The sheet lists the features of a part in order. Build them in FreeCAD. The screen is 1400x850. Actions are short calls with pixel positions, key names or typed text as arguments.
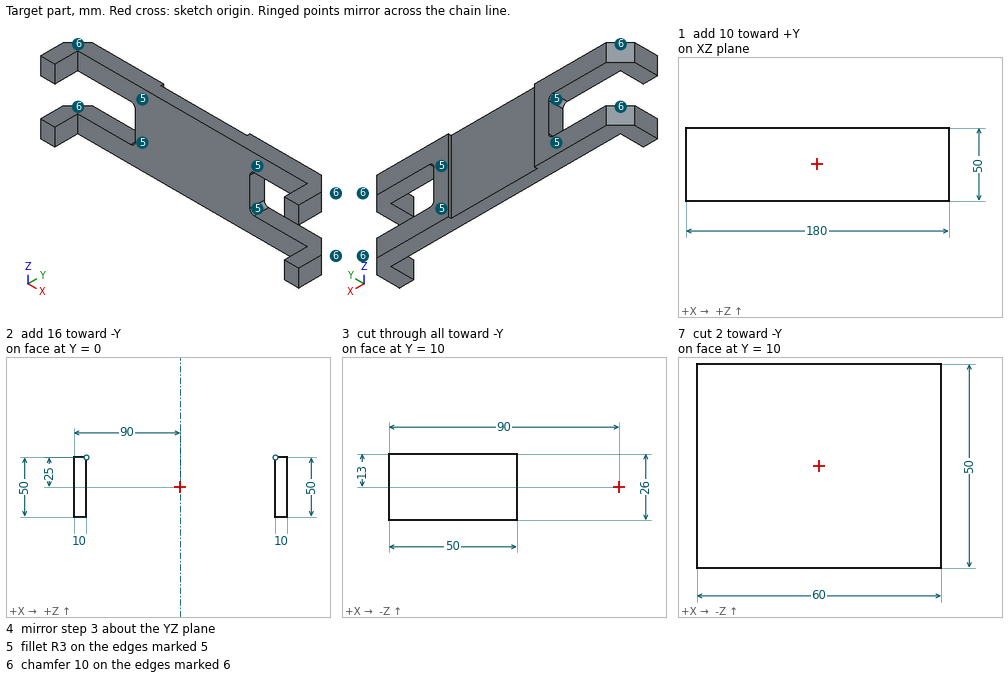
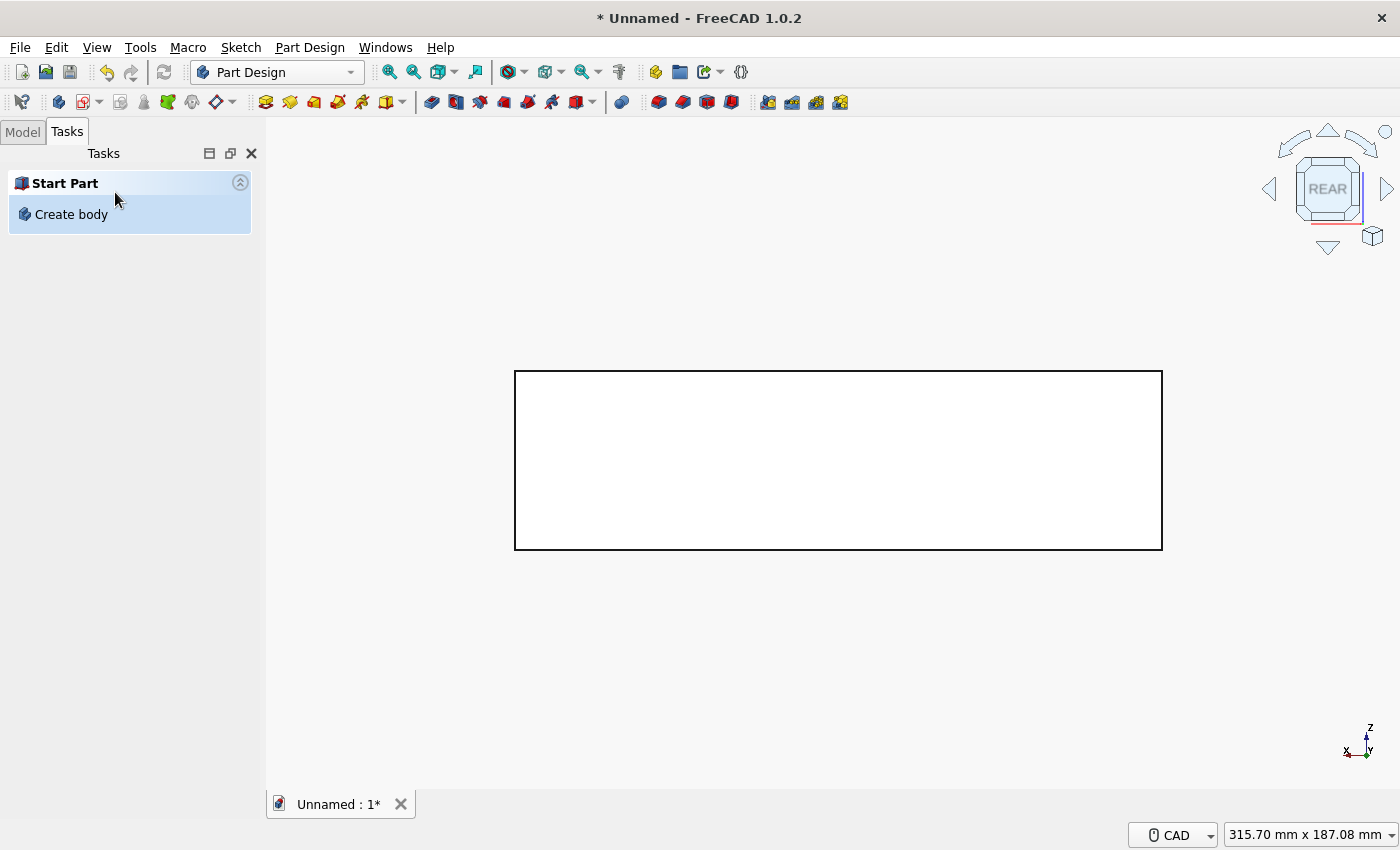
click(654, 459)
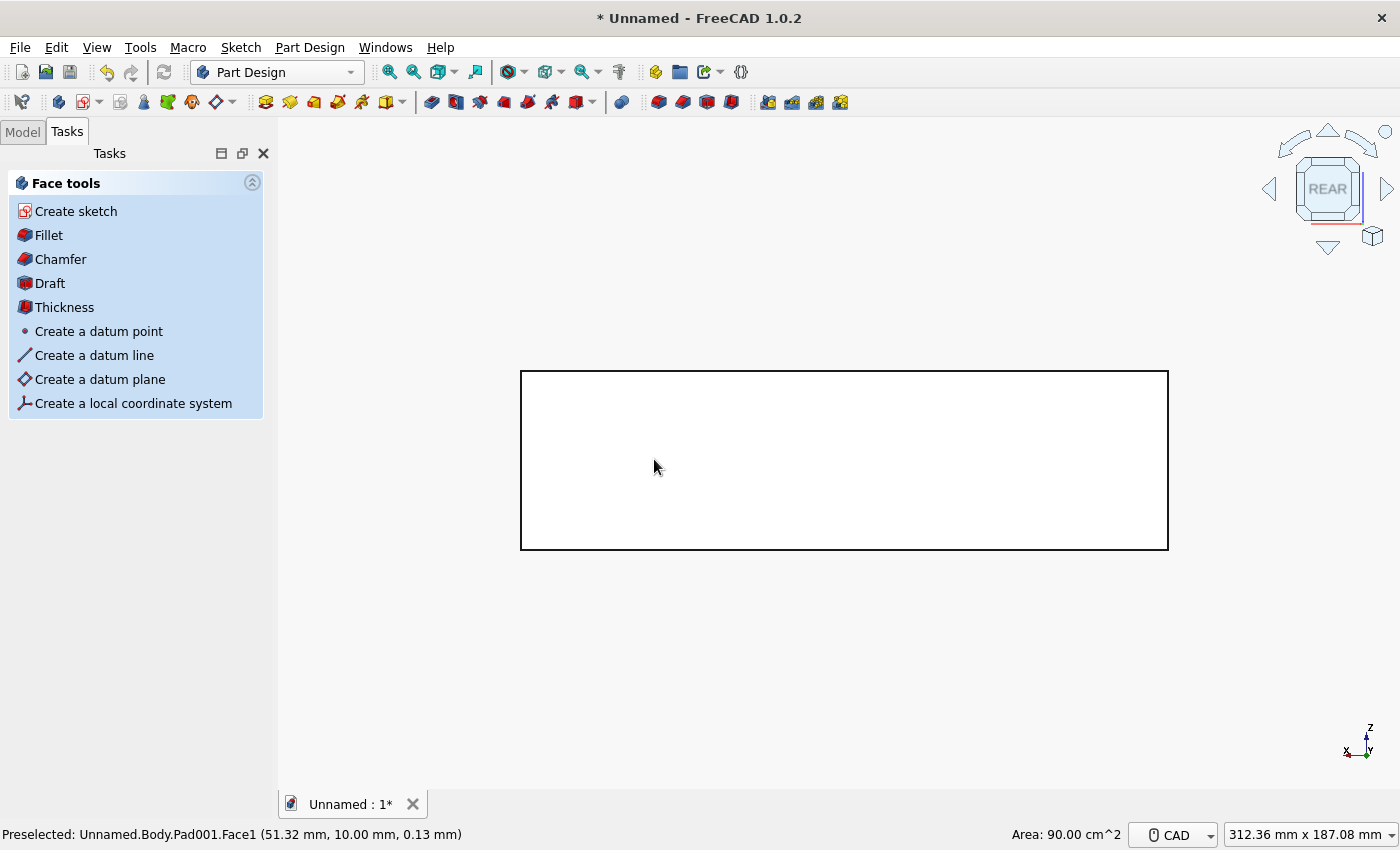
click(84, 102)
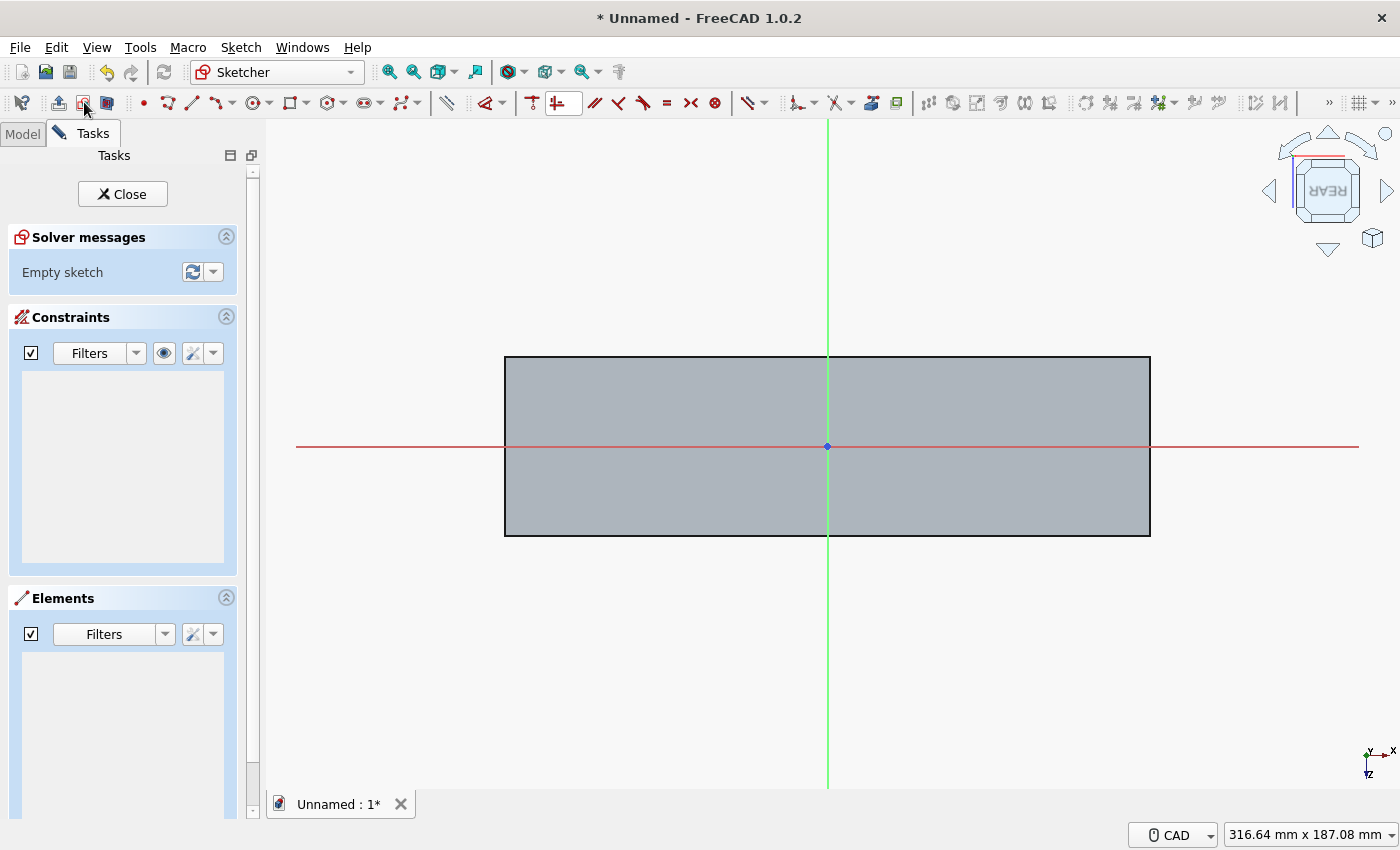
scroll(587, 440, up, 4)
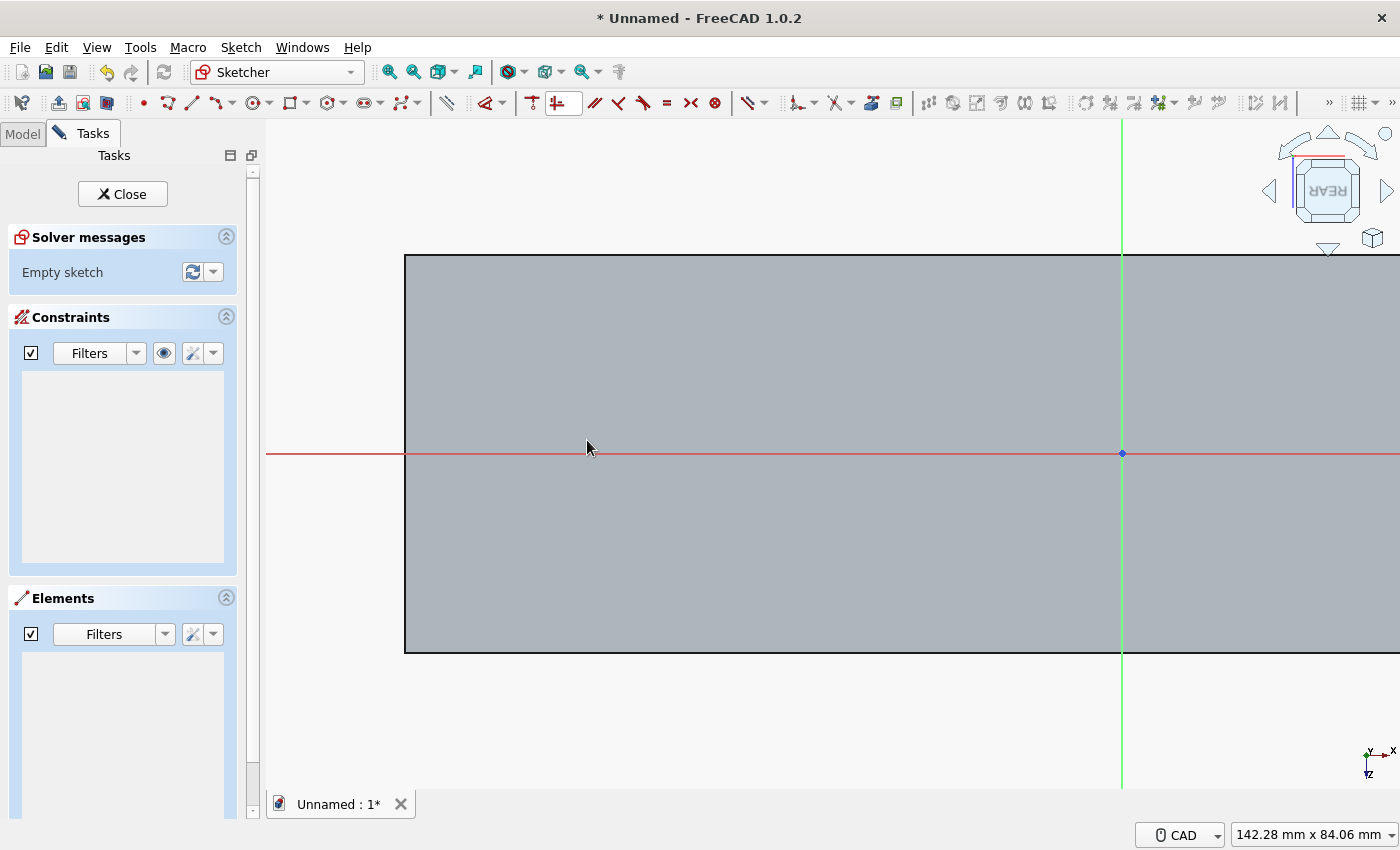
key(g)
key(r)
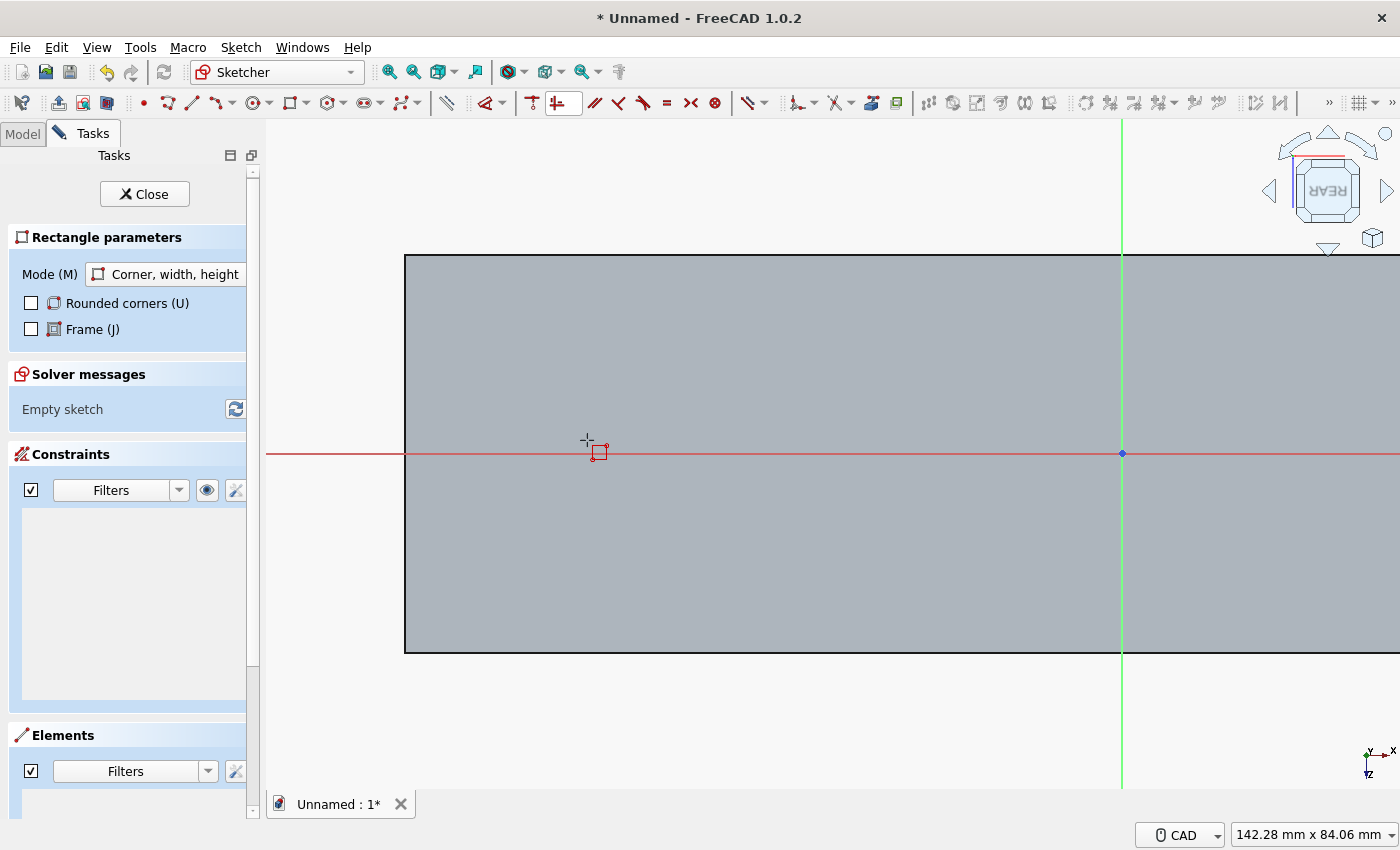
click(405, 350)
move(803, 558)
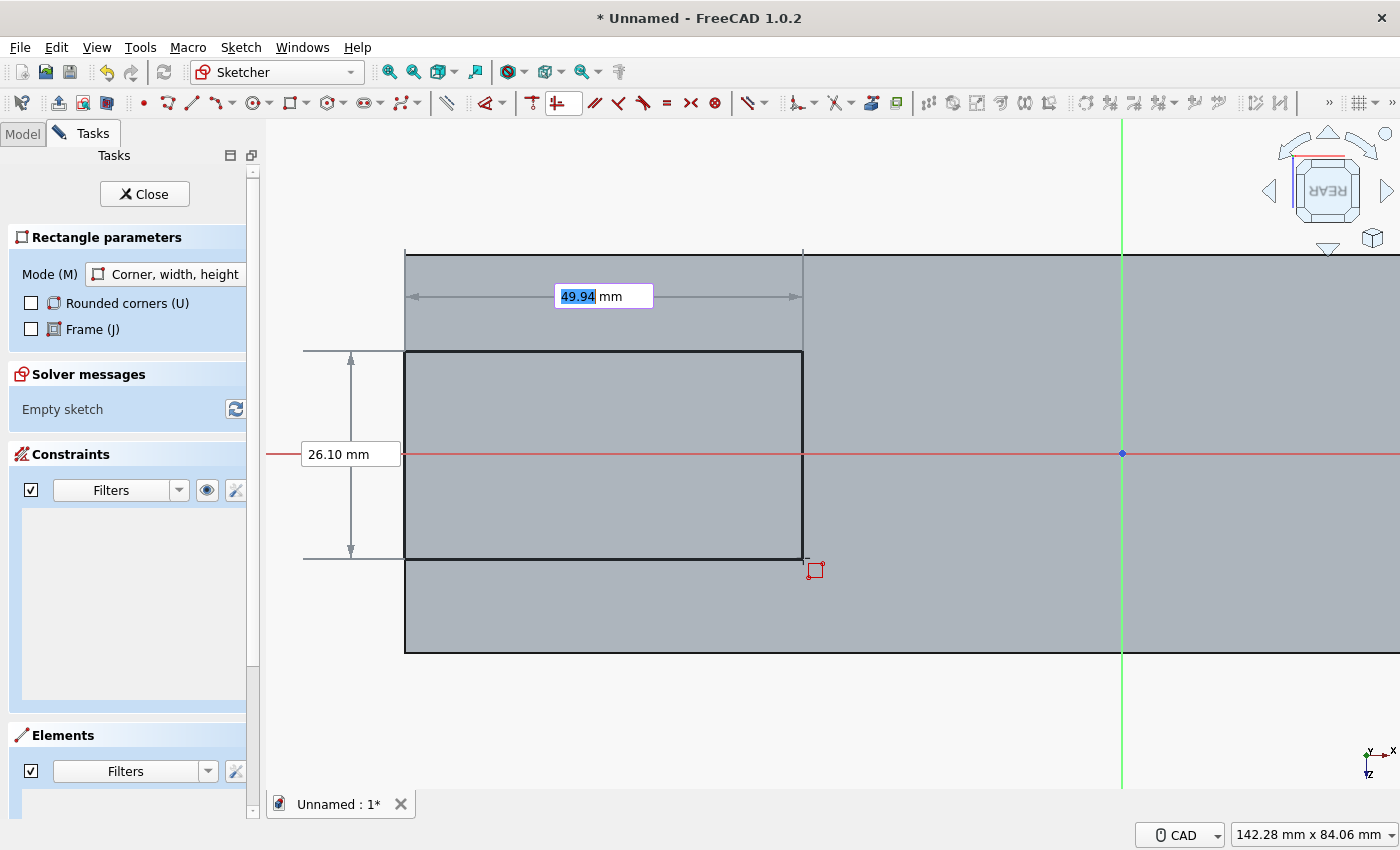
text(50)
key(Tab)
text(26)
key(Return)
key(Escape)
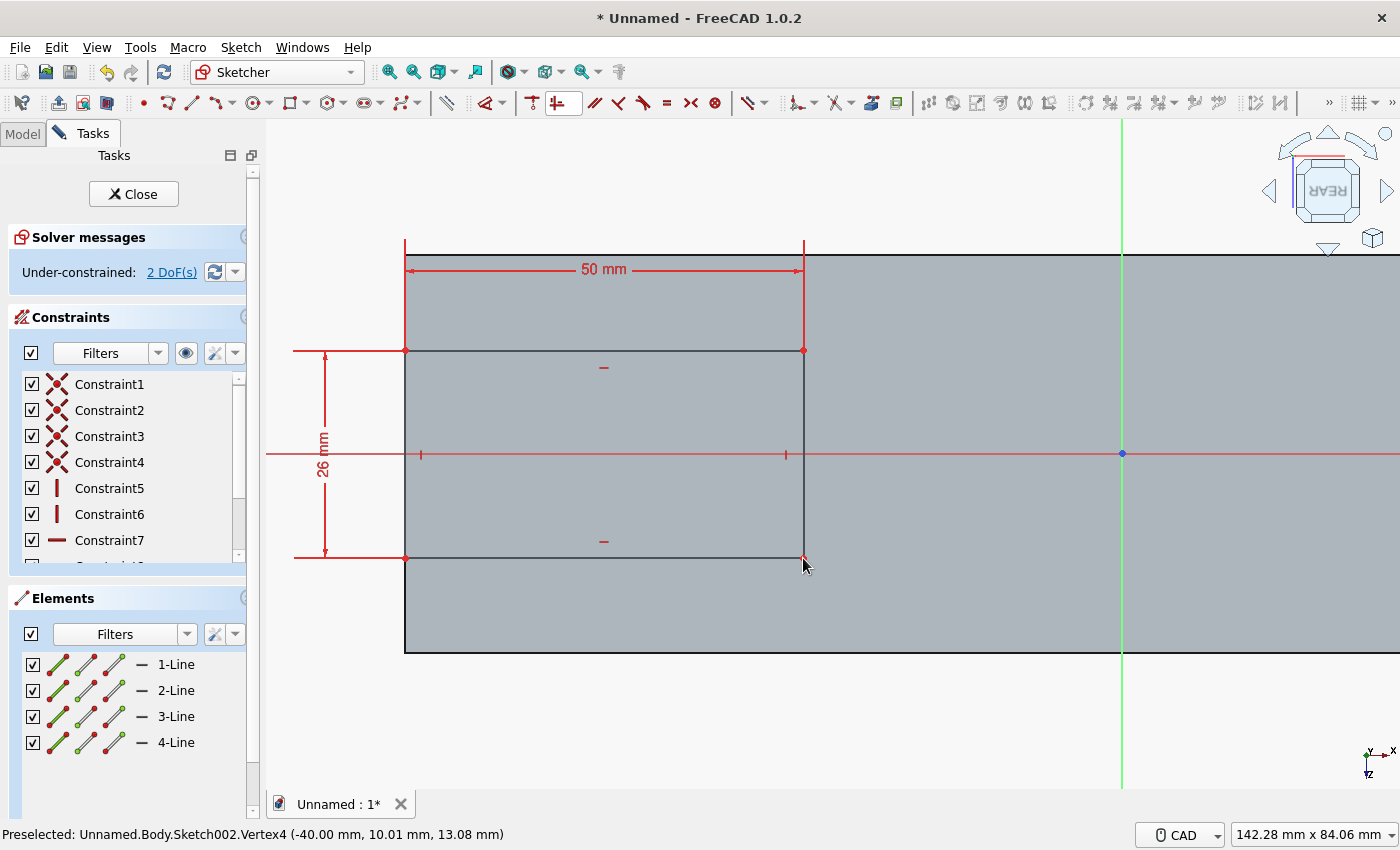
click(405, 351)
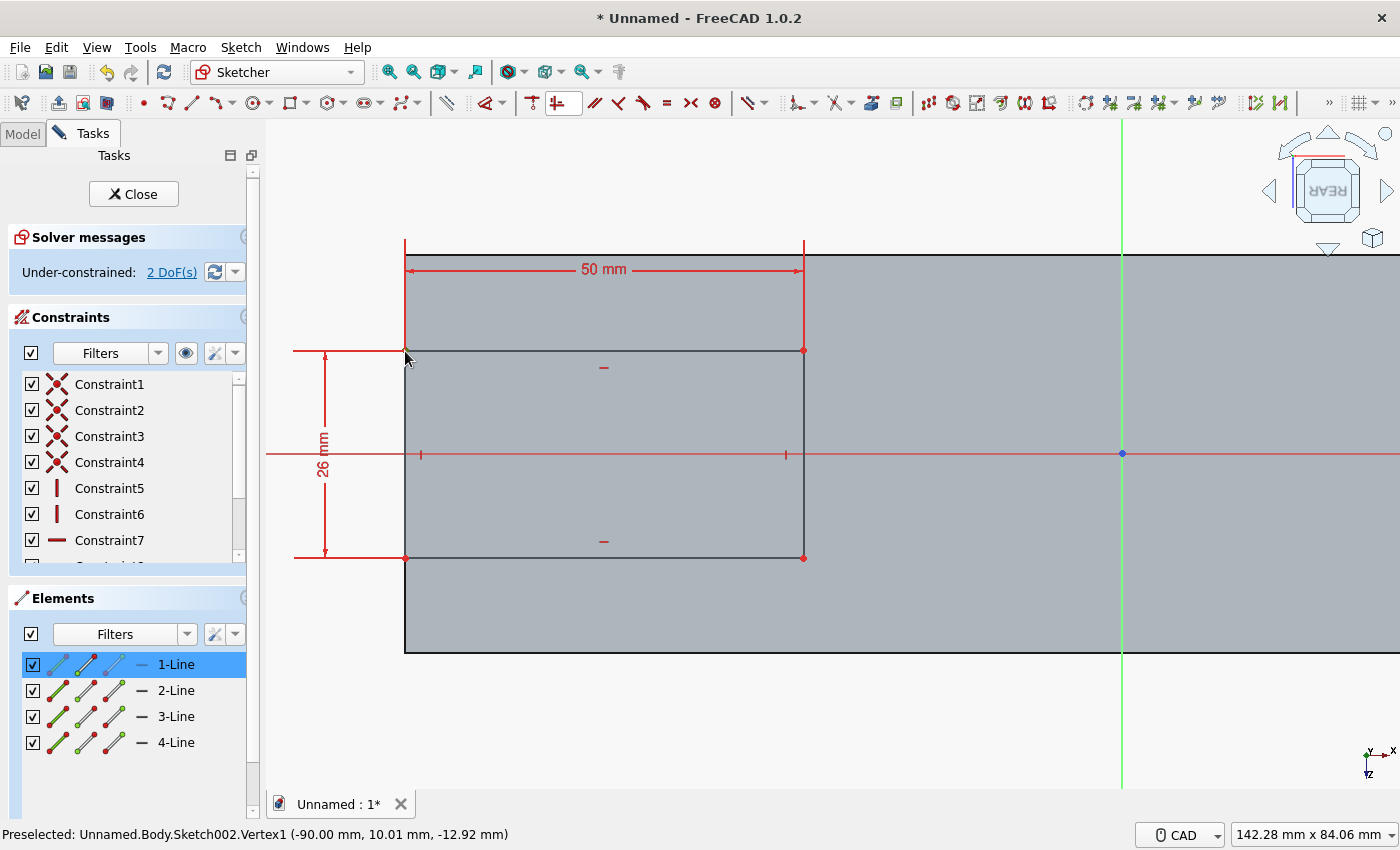
click(504, 104)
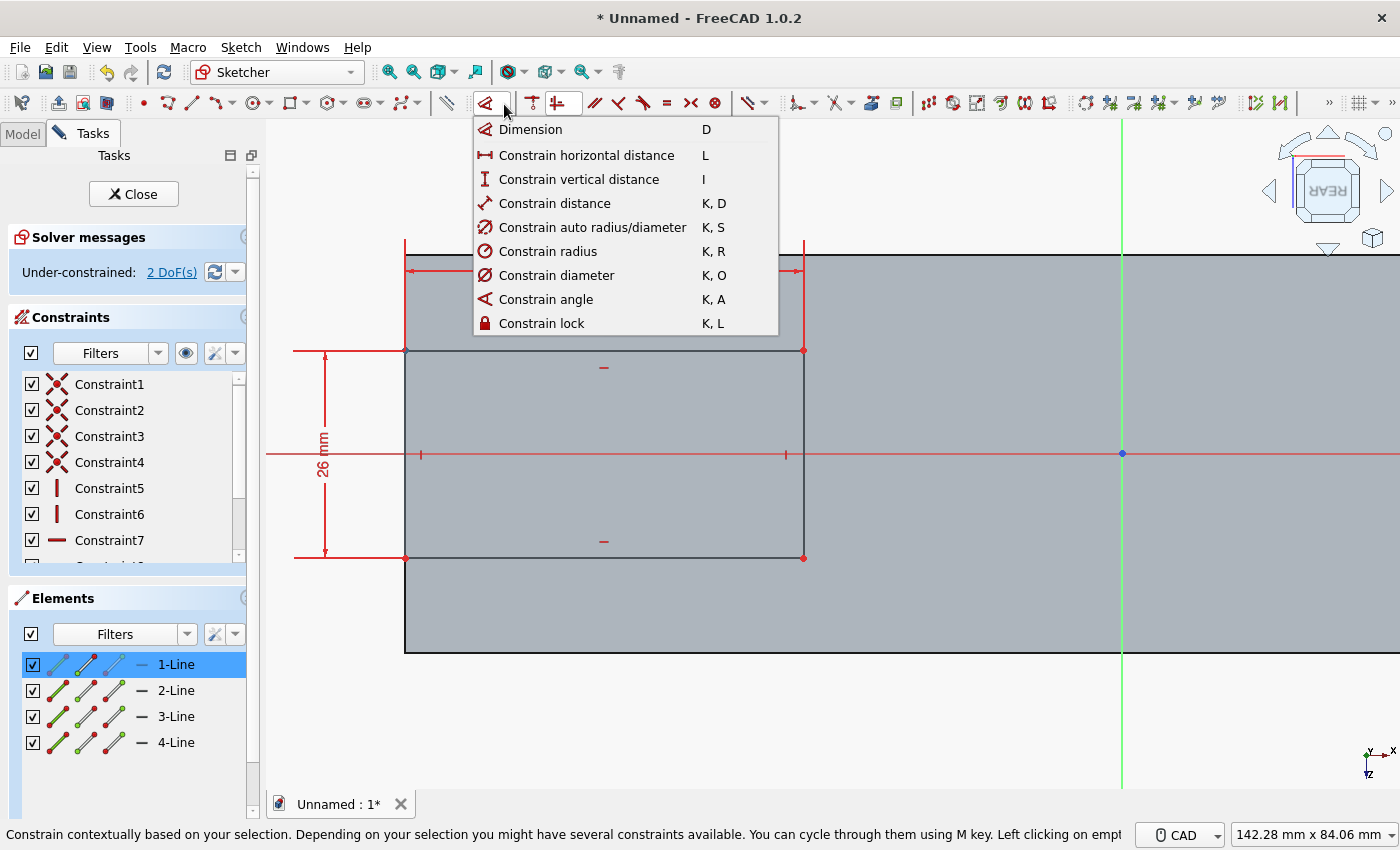
click(626, 155)